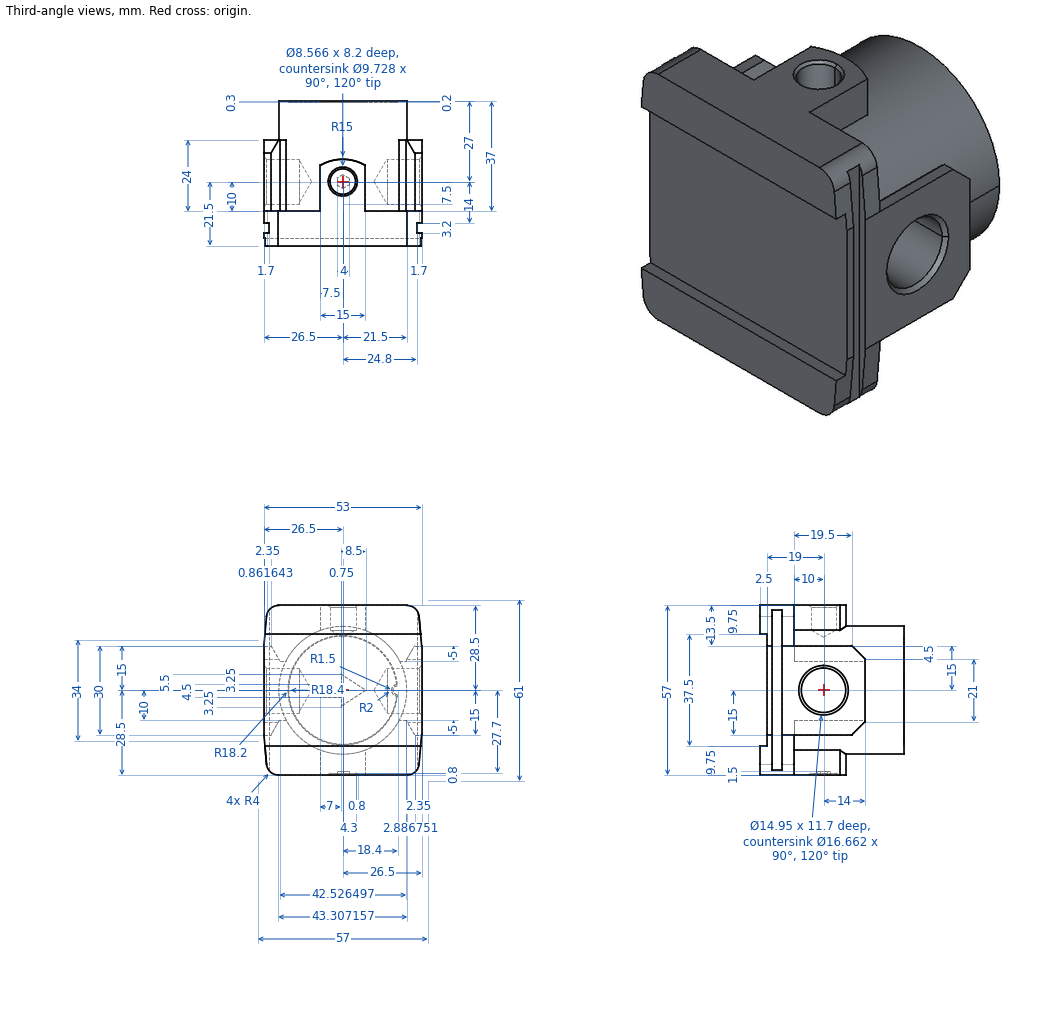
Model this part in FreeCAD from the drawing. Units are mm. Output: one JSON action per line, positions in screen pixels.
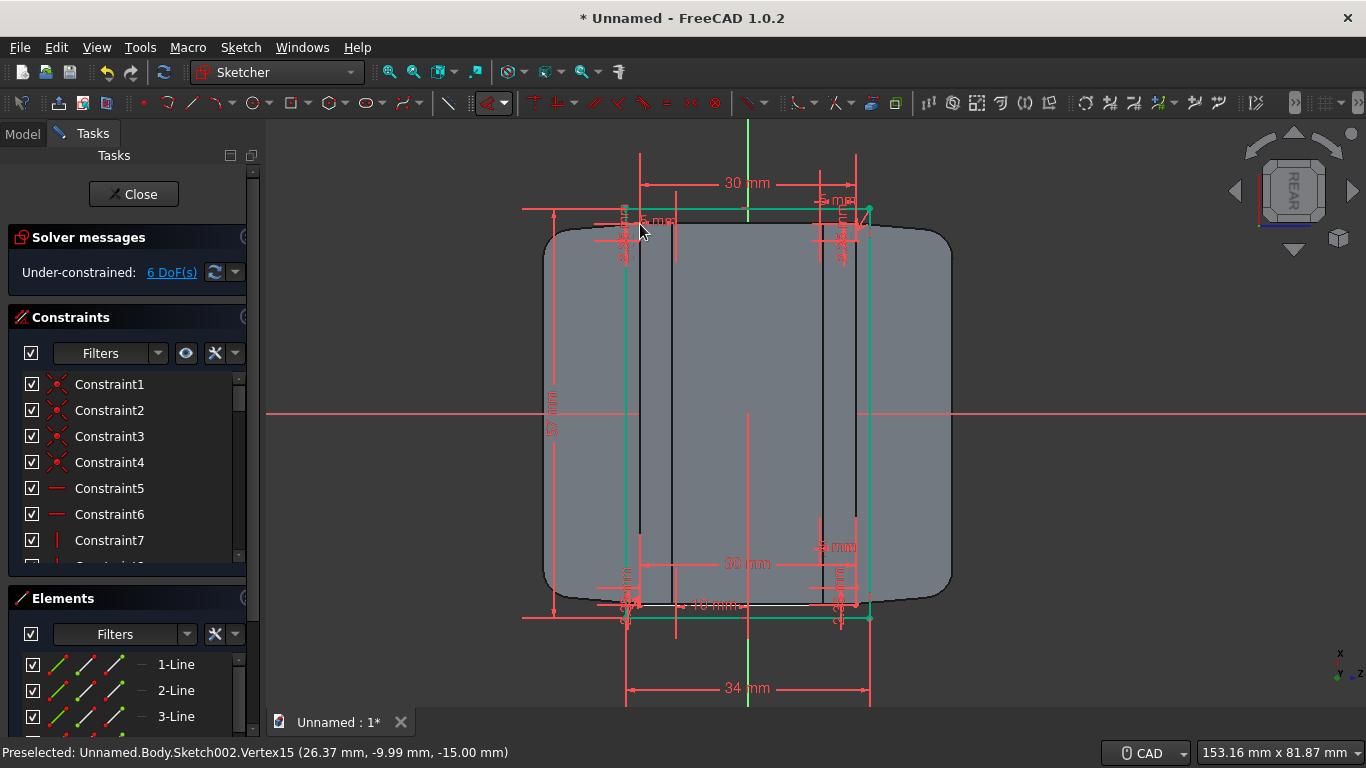
{"action": "left_click", "coordinate": [506, 104]}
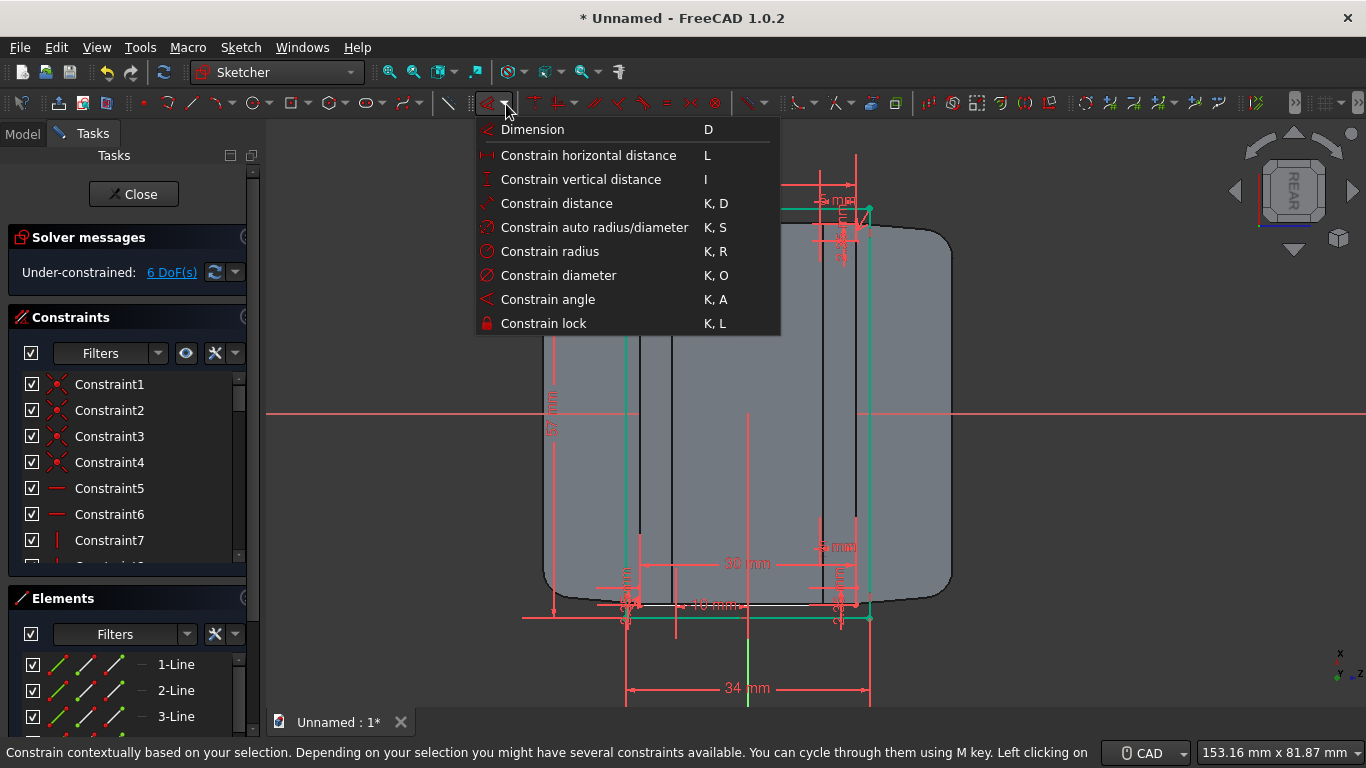
{"action": "left_click", "coordinate": [628, 179]}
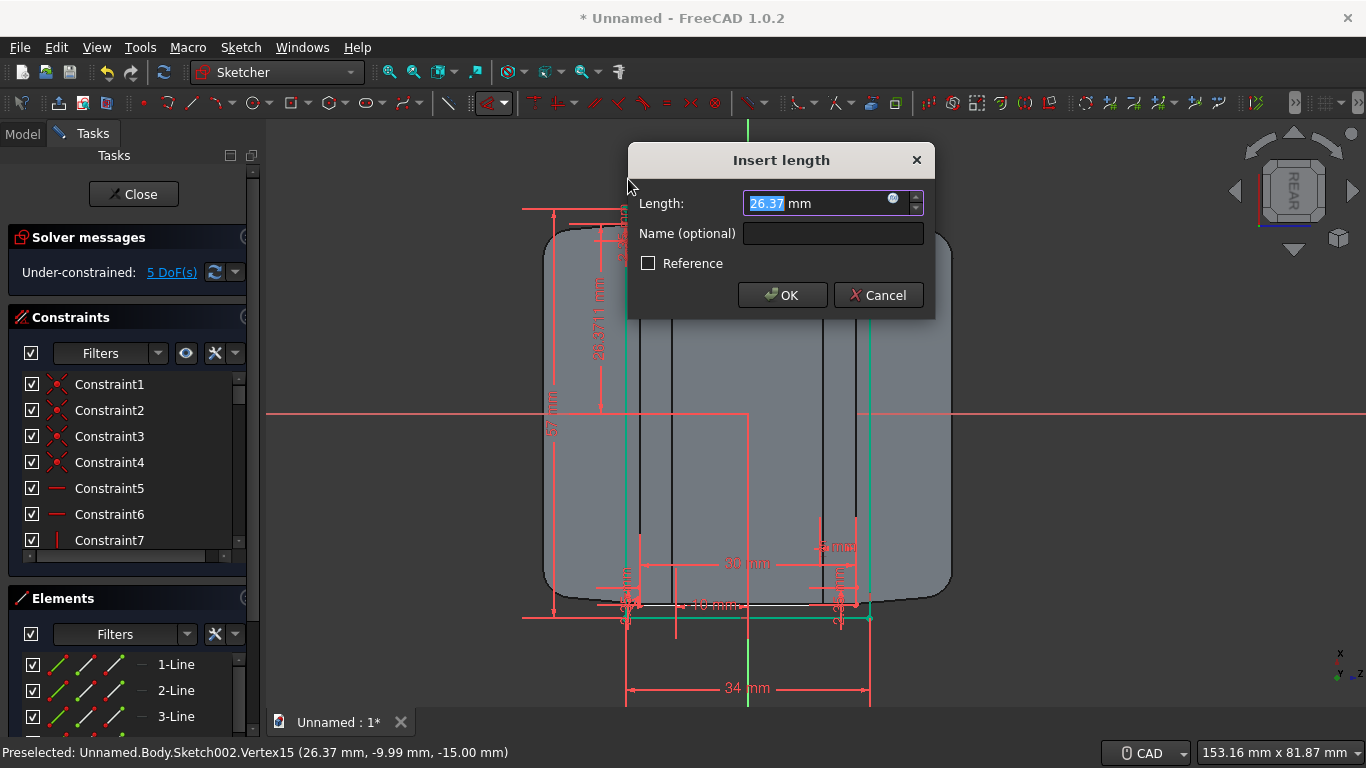
{"action": "type", "text": "26.5"}
{"action": "key", "text": "Return"}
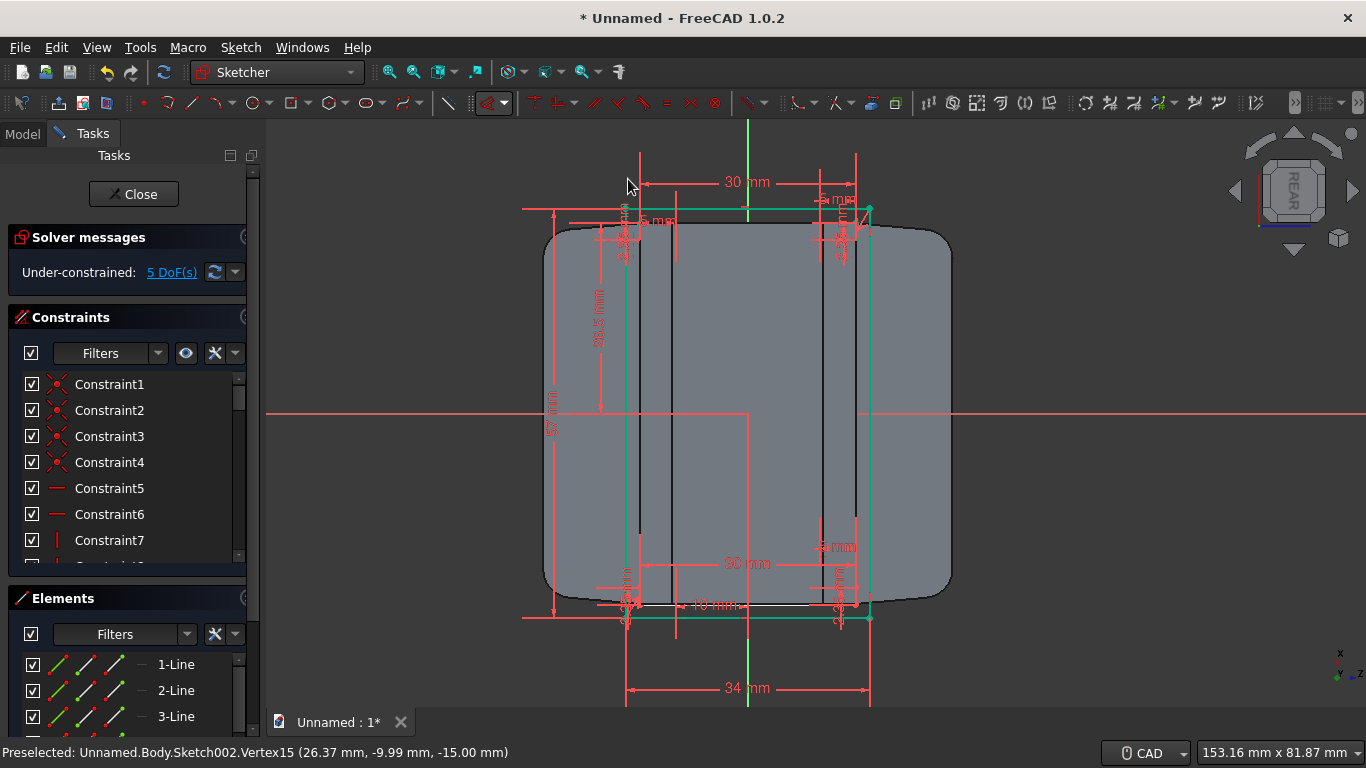
{"action": "left_click", "coordinate": [856, 605]}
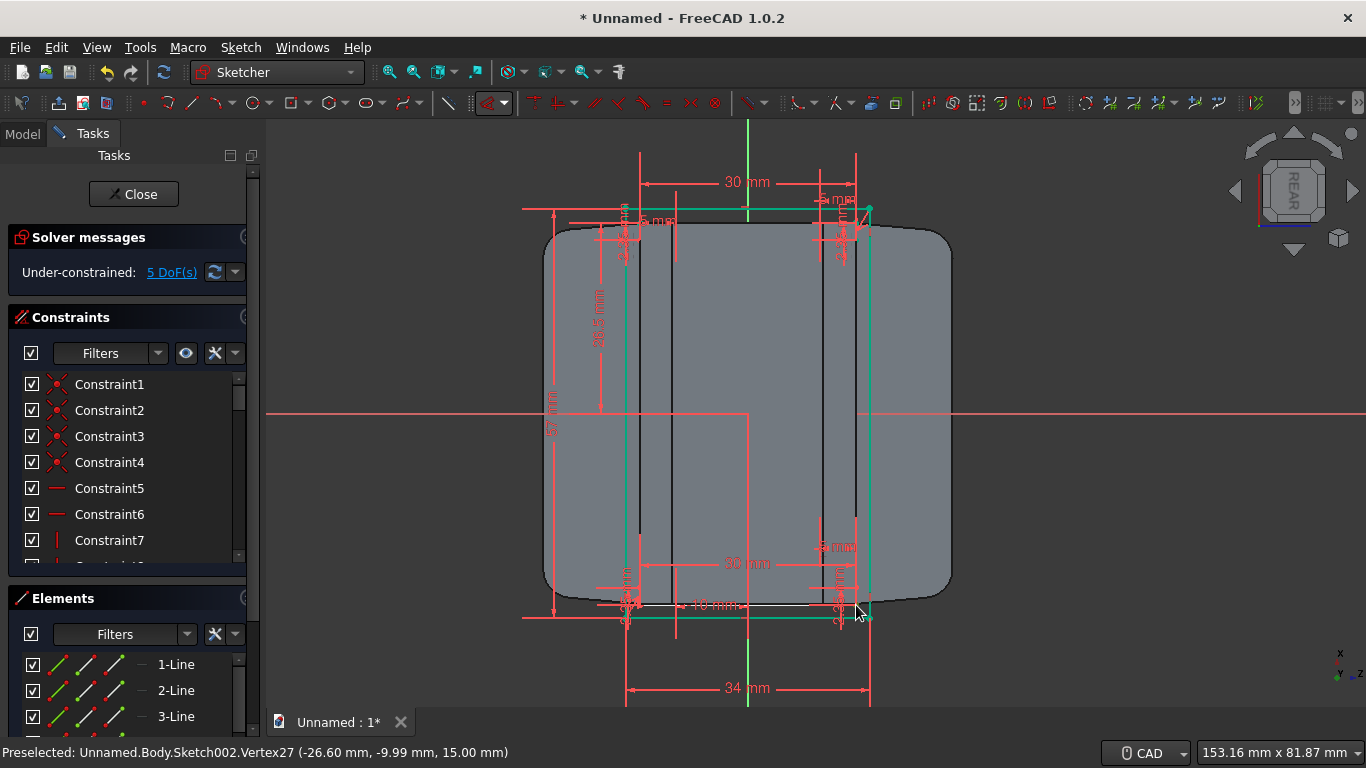
{"action": "key", "text": "i"}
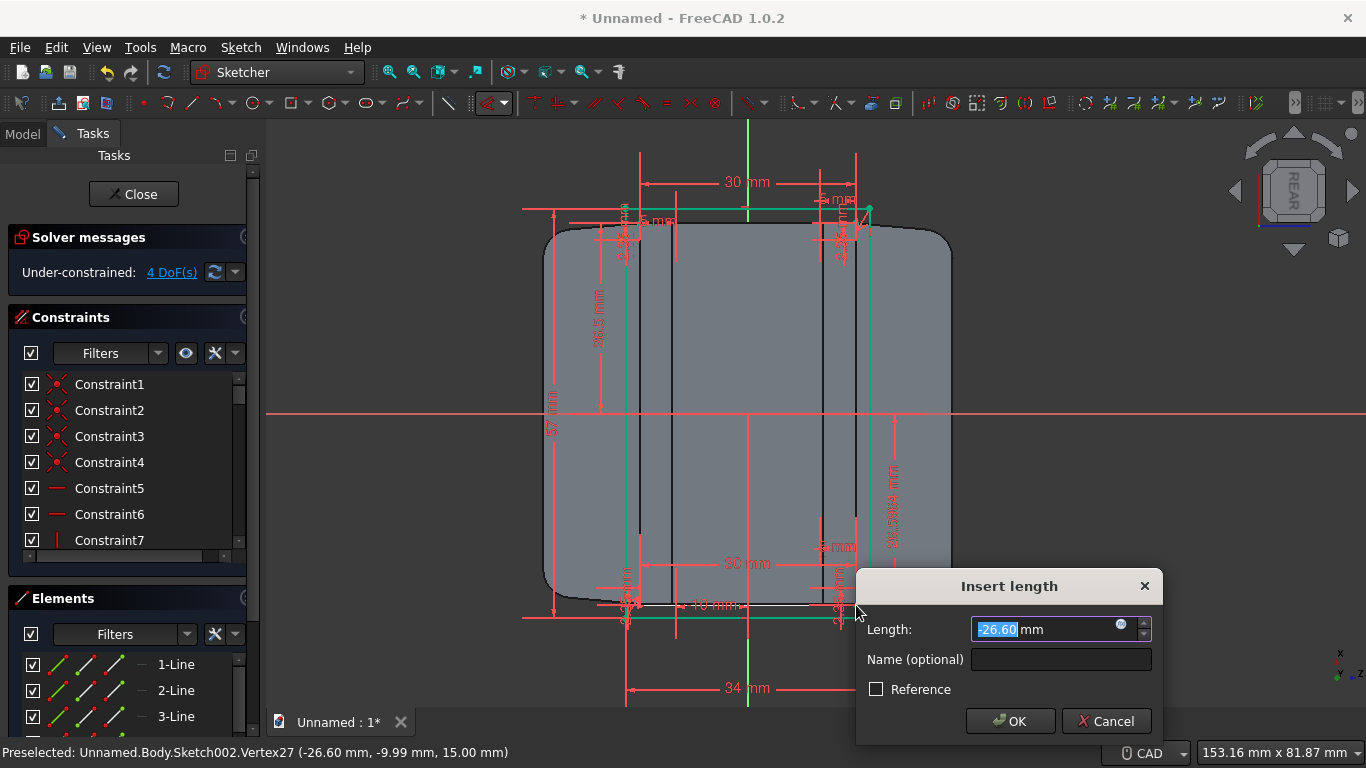
{"action": "type", "text": "-26.5"}
{"action": "key", "text": "Return"}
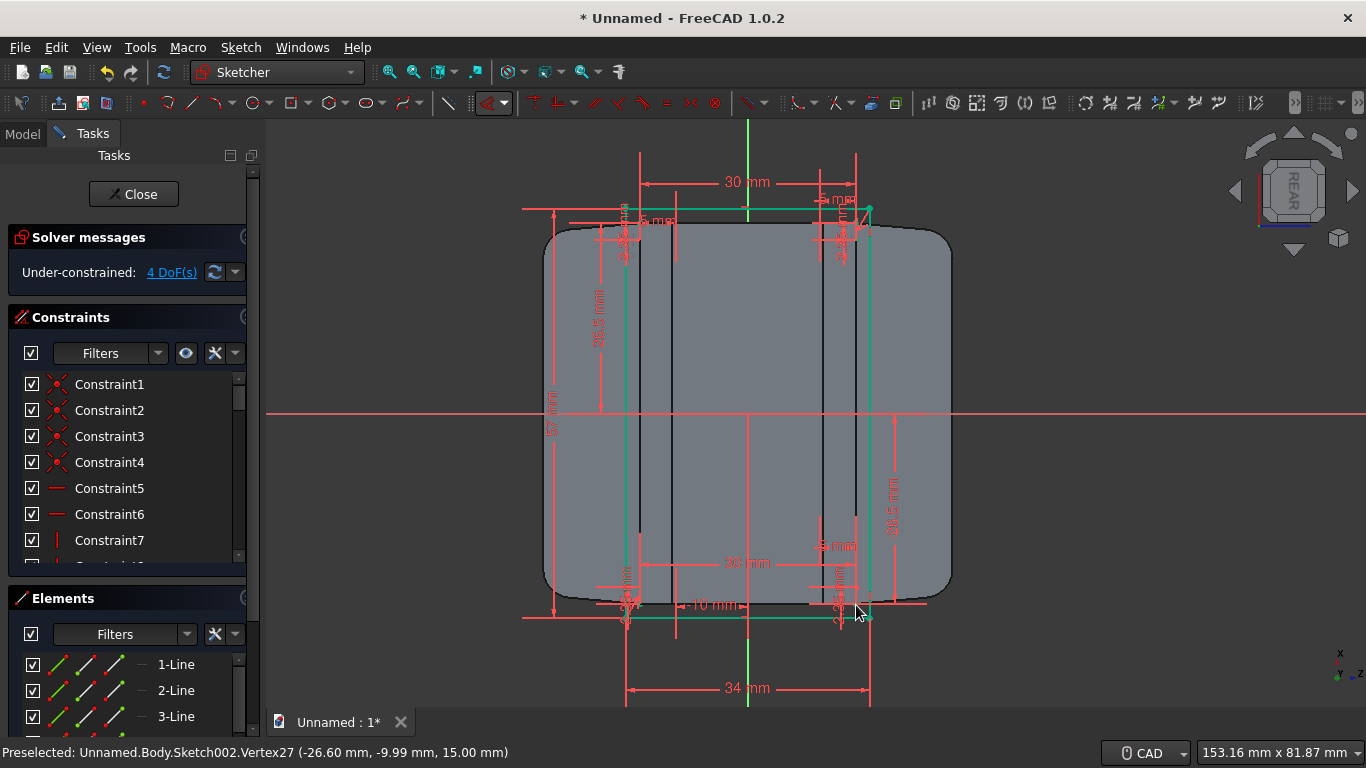
{"action": "left_click", "coordinate": [676, 476]}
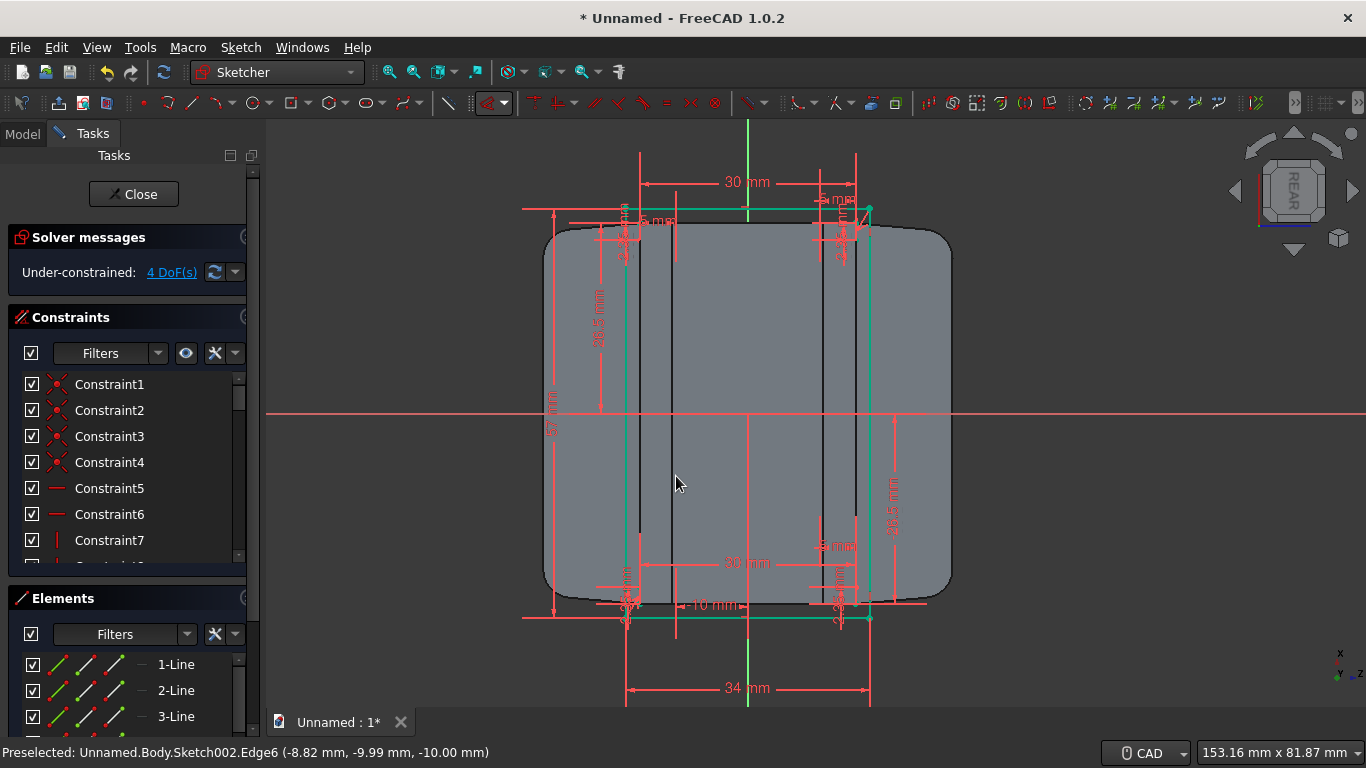
{"action": "left_click", "coordinate": [506, 104]}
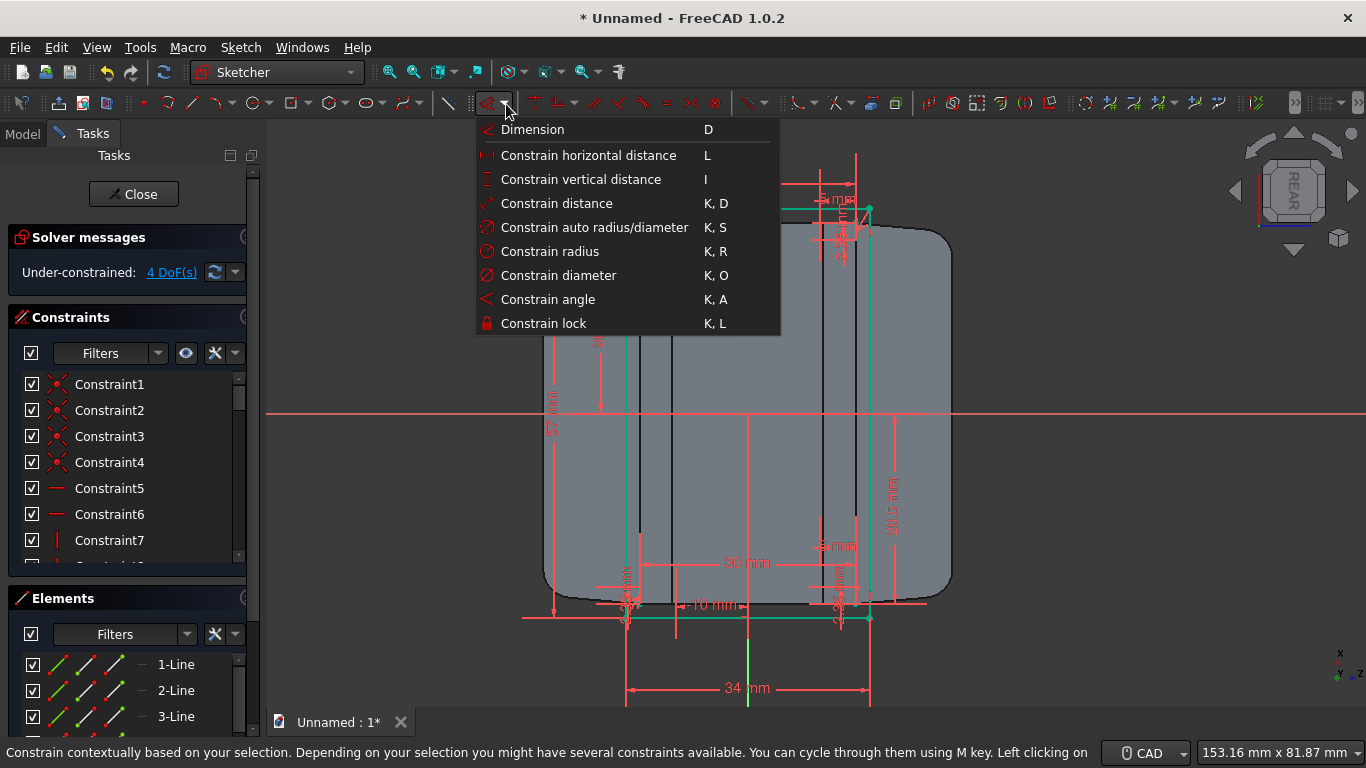
{"action": "left_click", "coordinate": [628, 179]}